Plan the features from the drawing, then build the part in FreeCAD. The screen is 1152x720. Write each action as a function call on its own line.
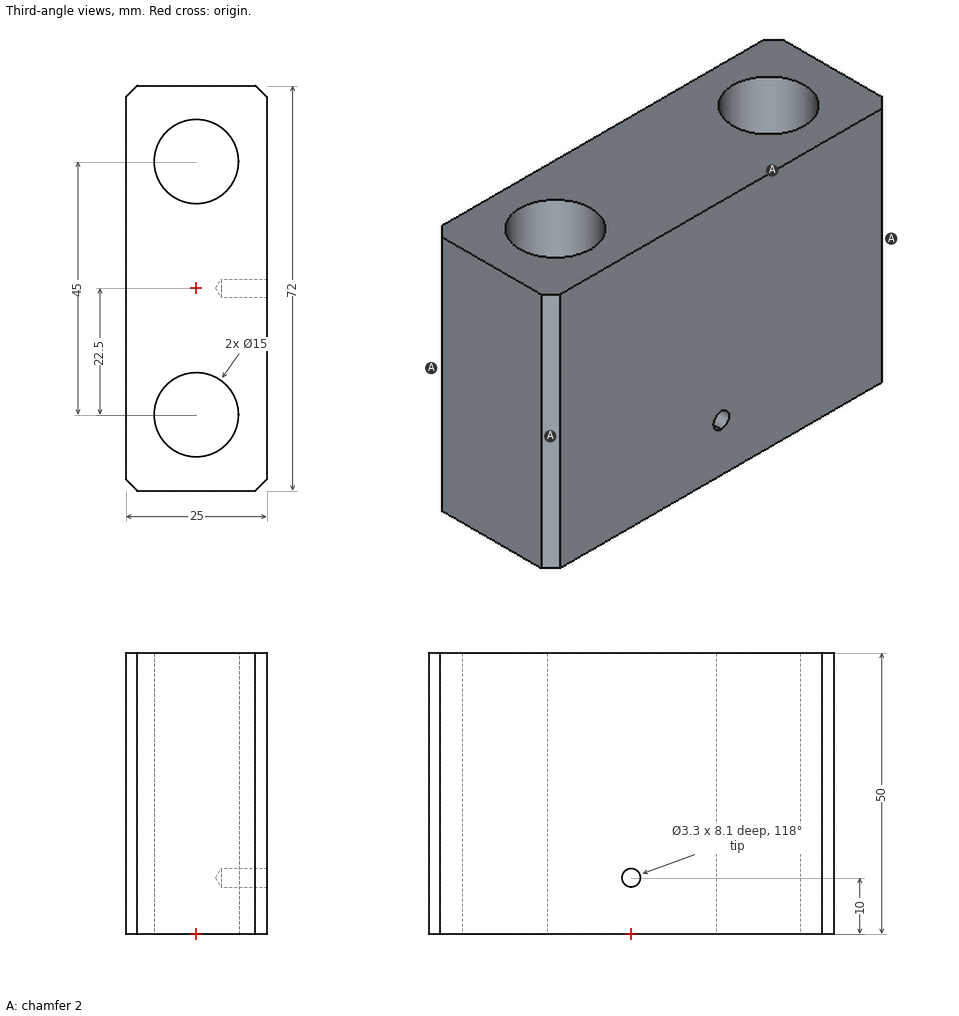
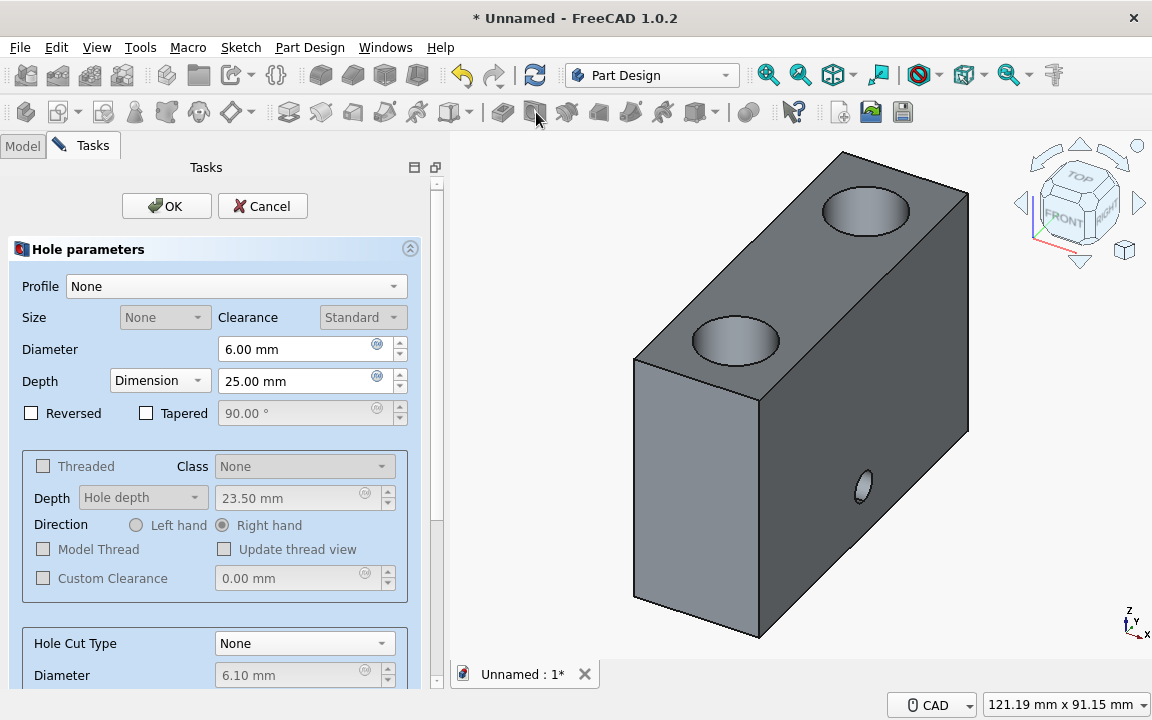
triple_click(305, 349)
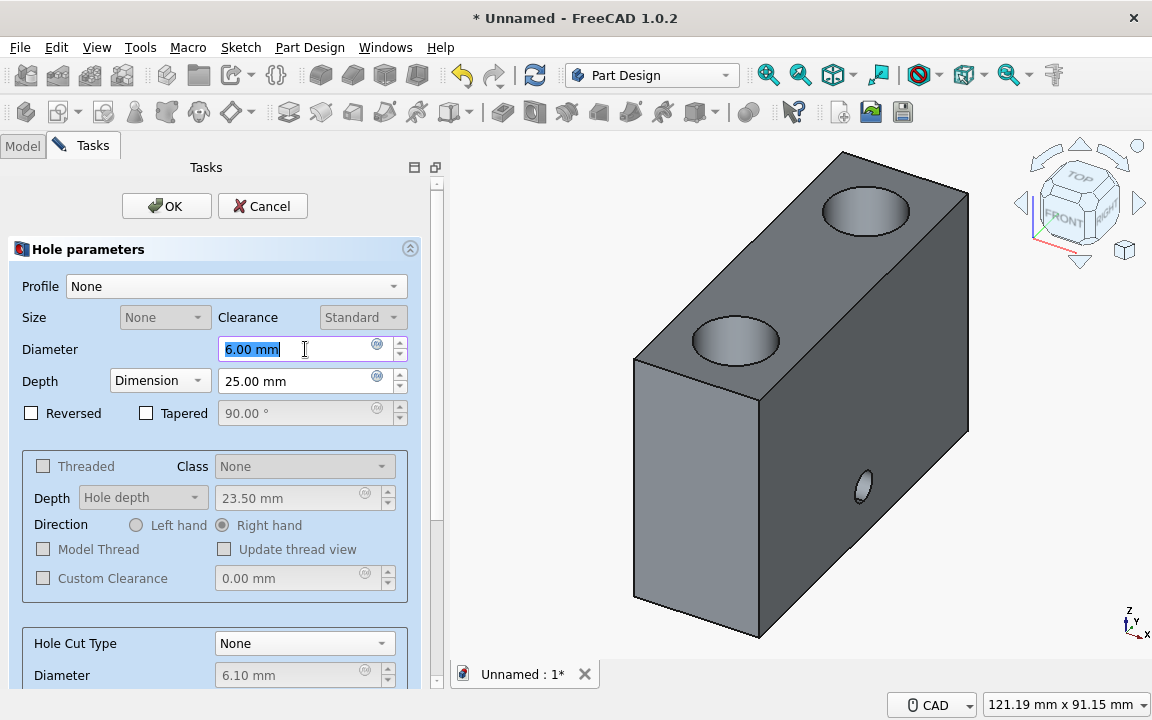
text(3.3)
key(Tab)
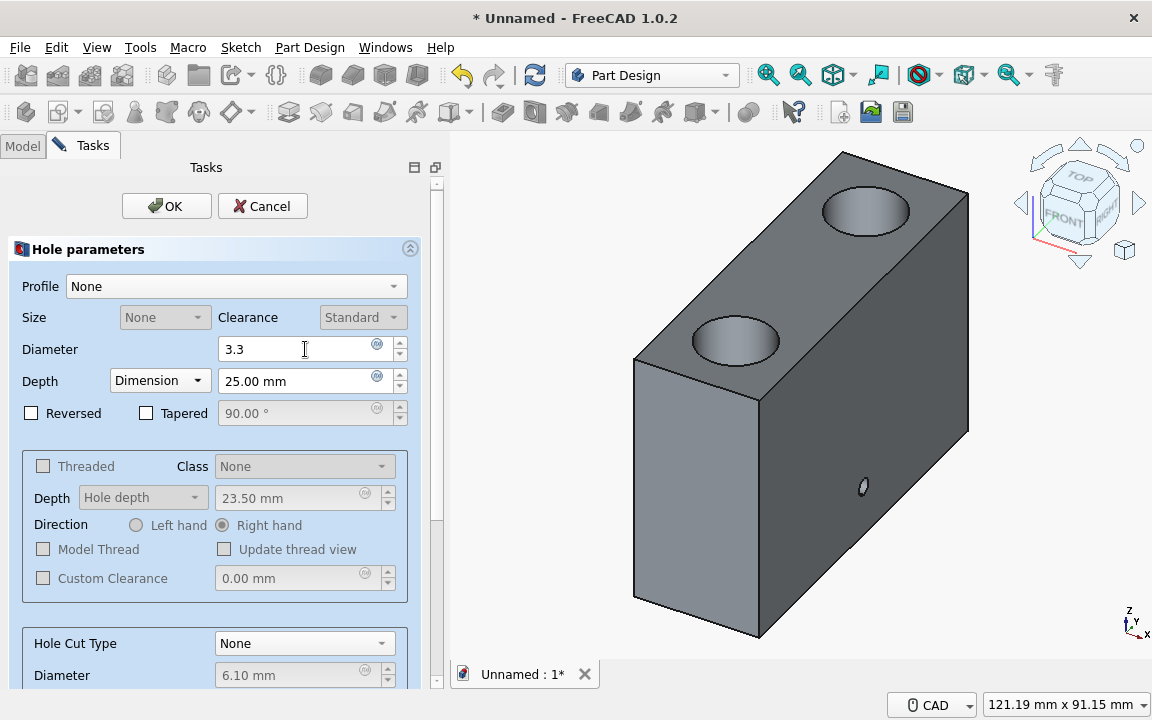
triple_click(305, 381)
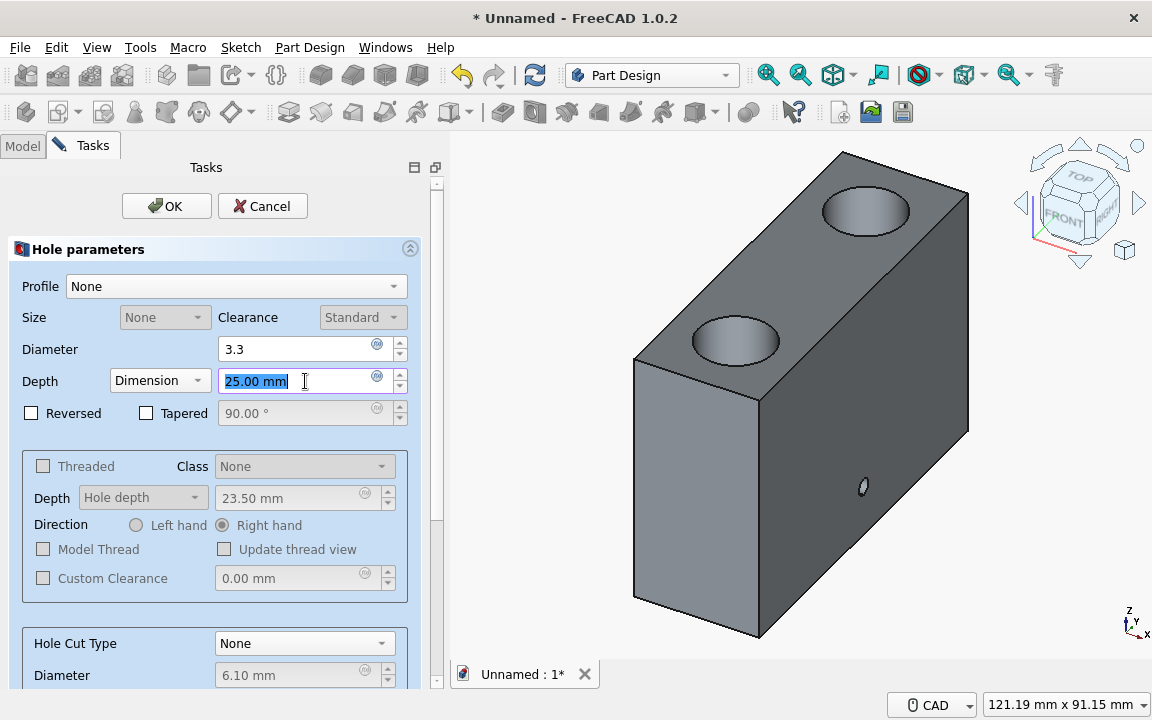
text(8.1)
key(Tab)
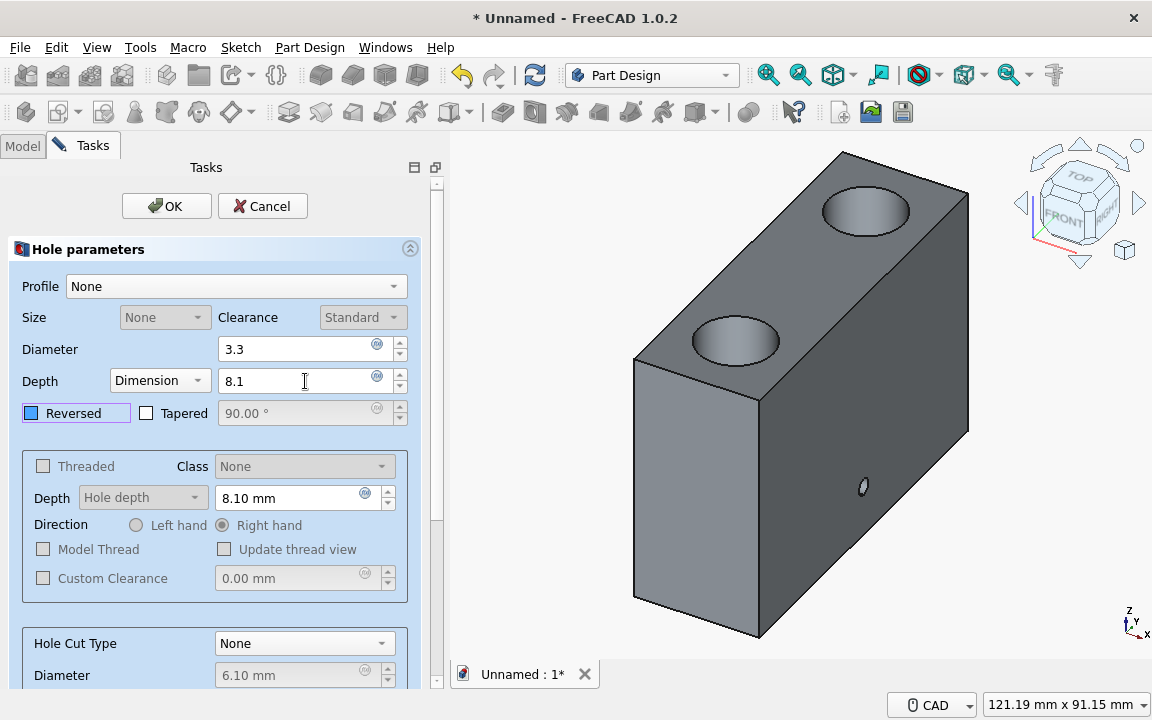
click(167, 206)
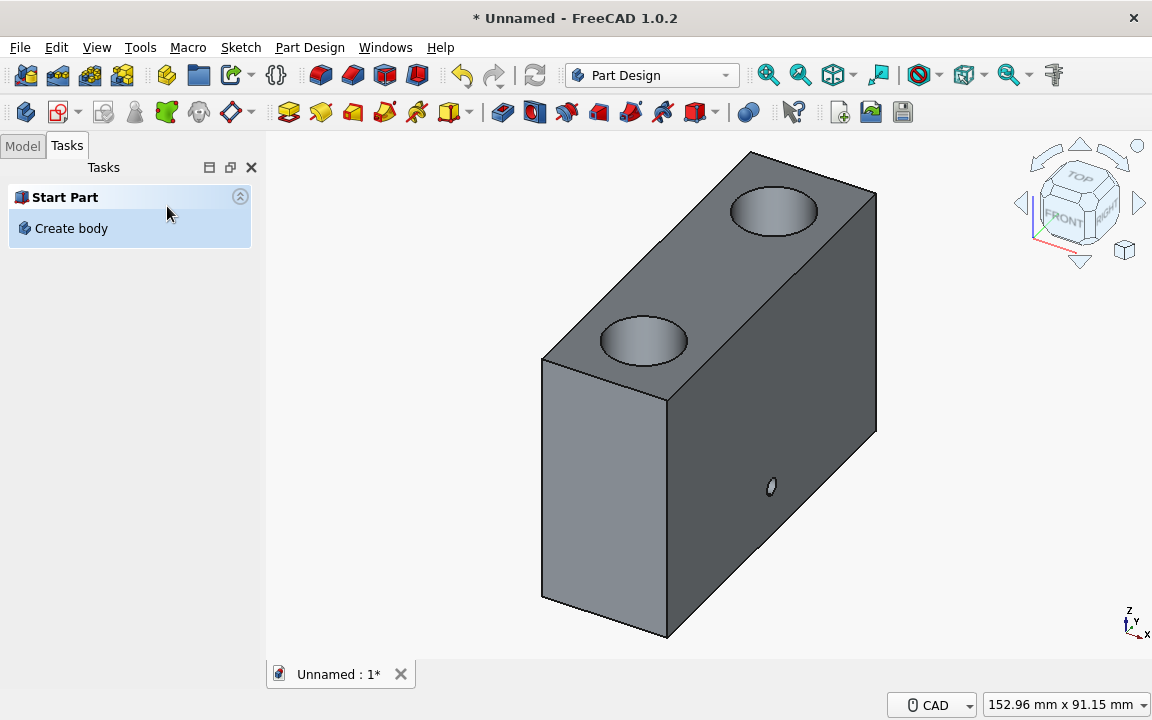
click(667, 518)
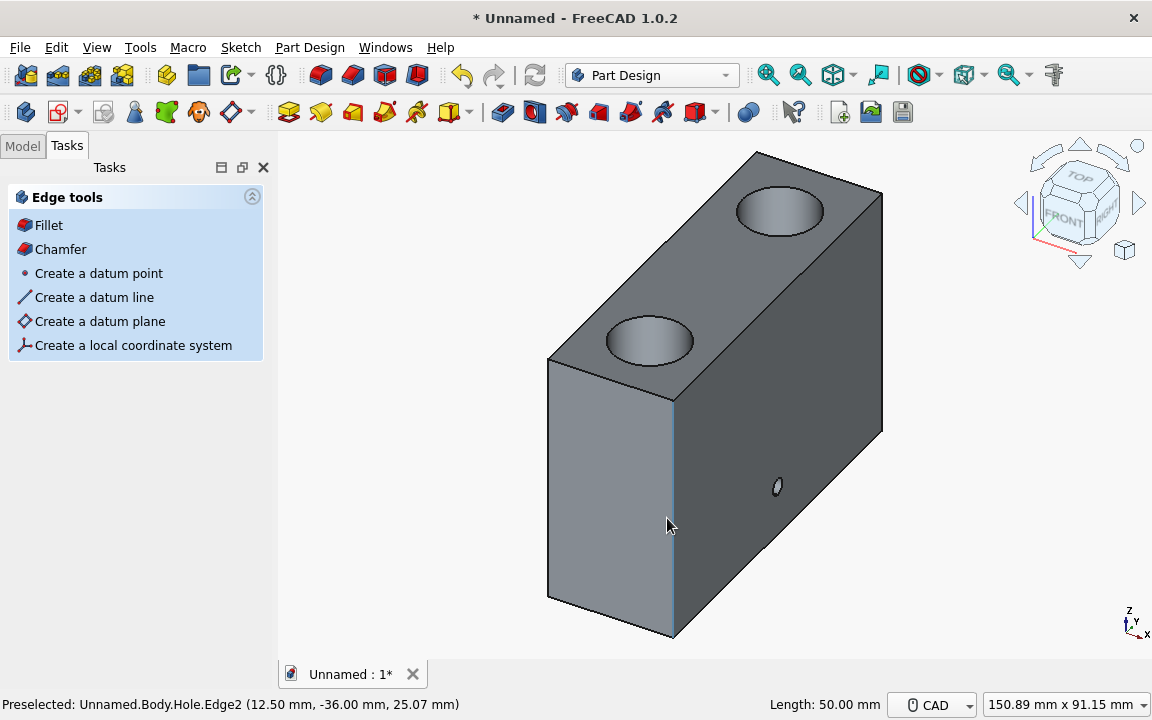
key(0)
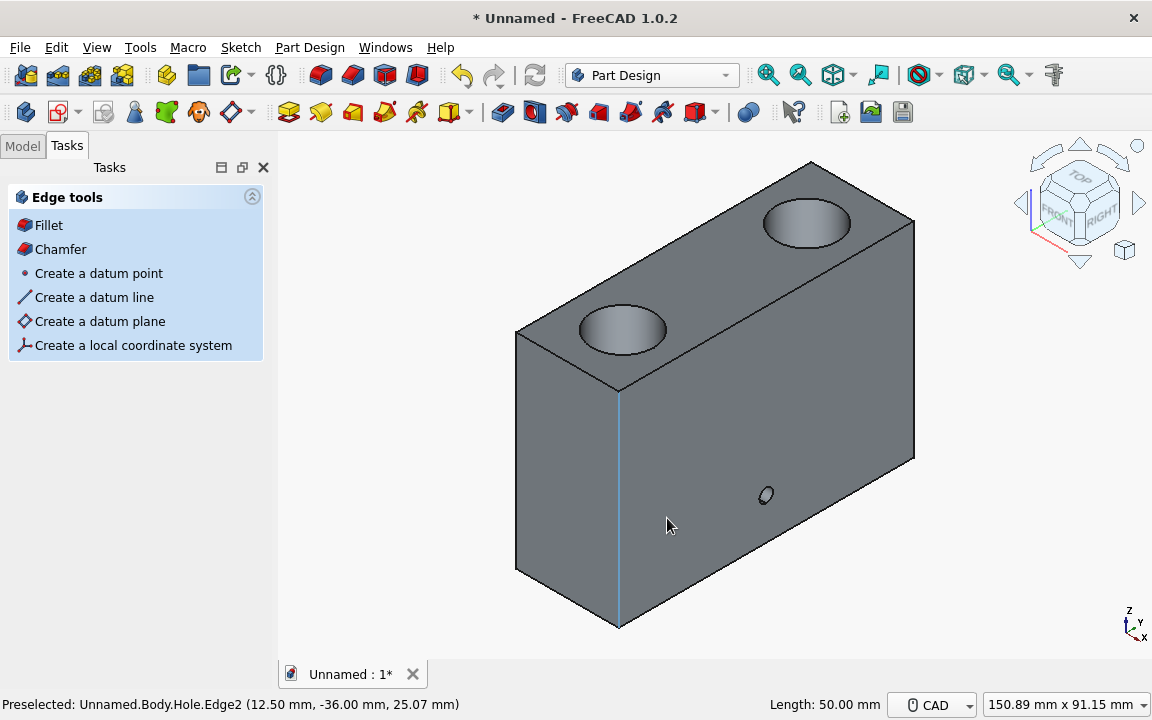
key(2)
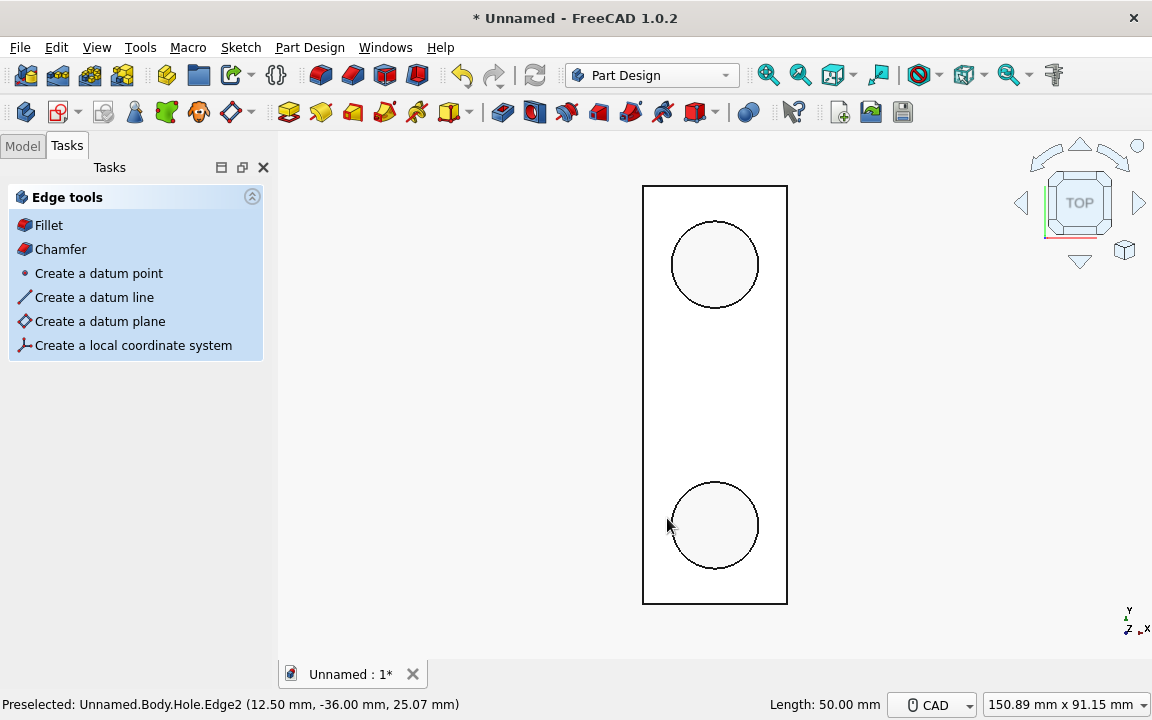
key(1)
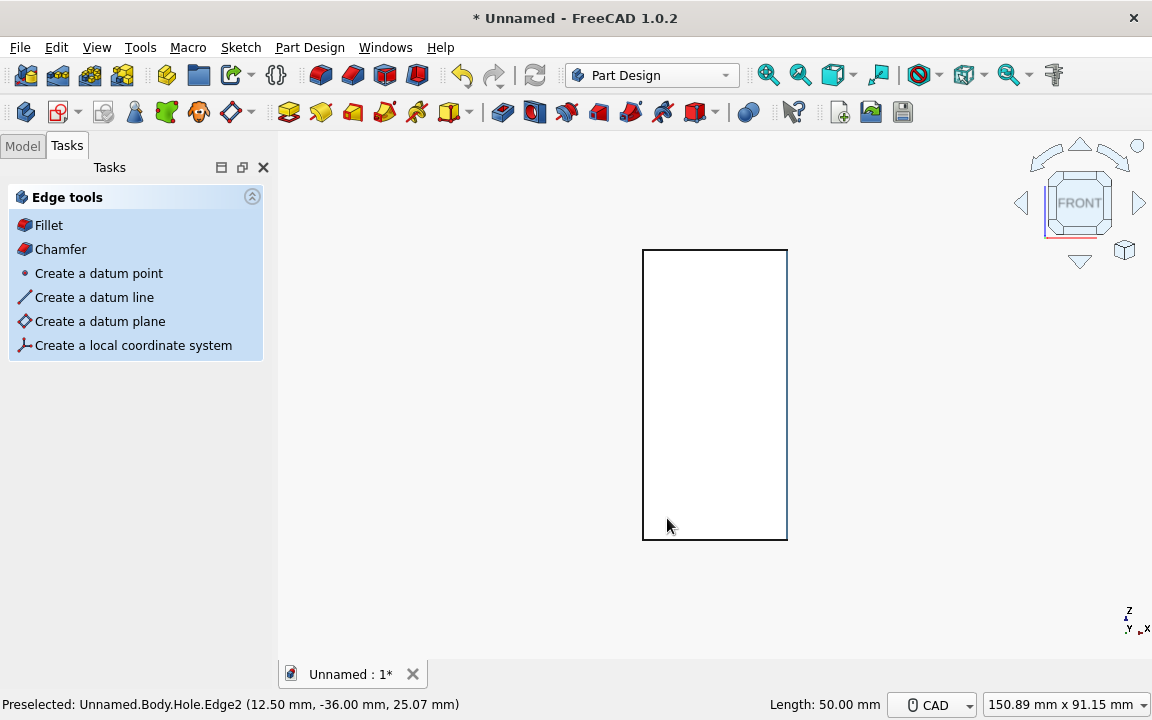
click(643, 394, ctrl)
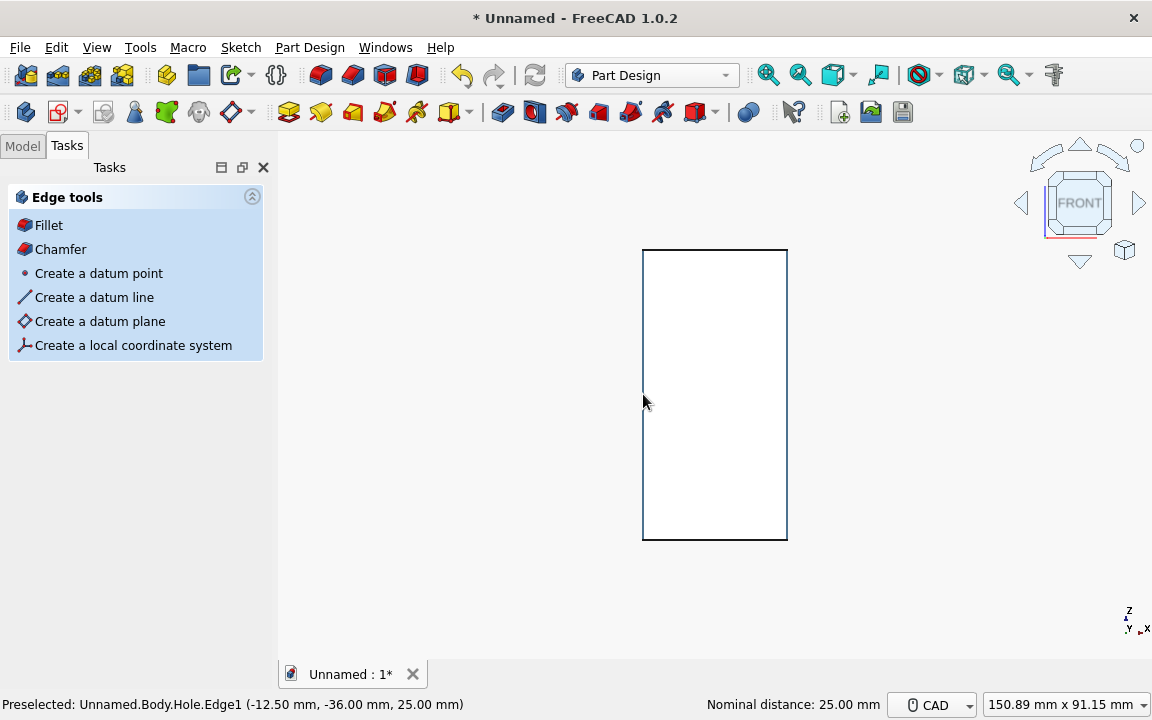
key(3)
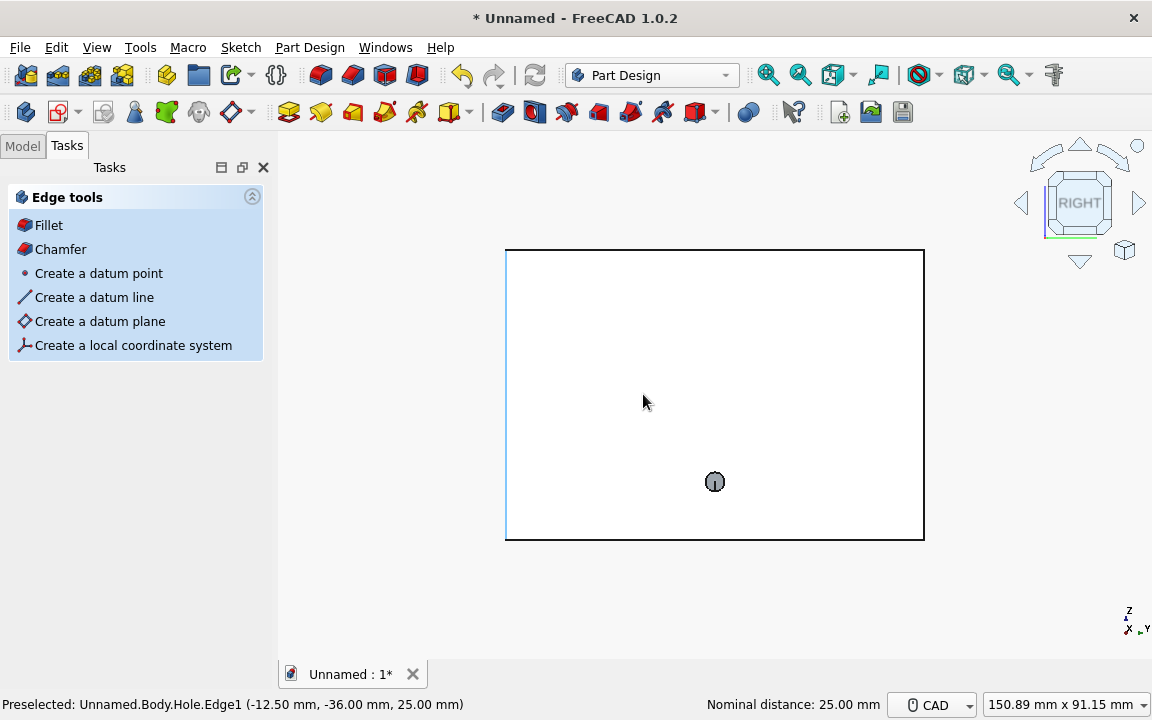
click(924, 394, ctrl)